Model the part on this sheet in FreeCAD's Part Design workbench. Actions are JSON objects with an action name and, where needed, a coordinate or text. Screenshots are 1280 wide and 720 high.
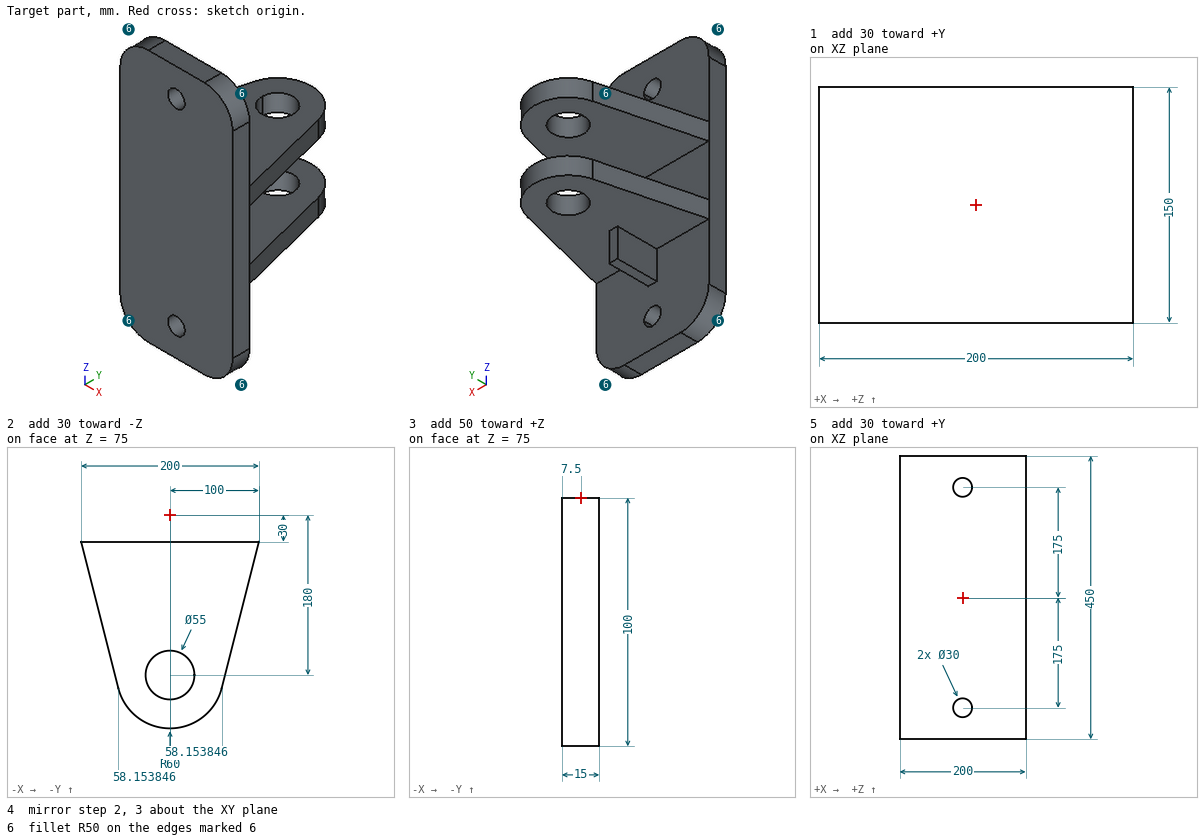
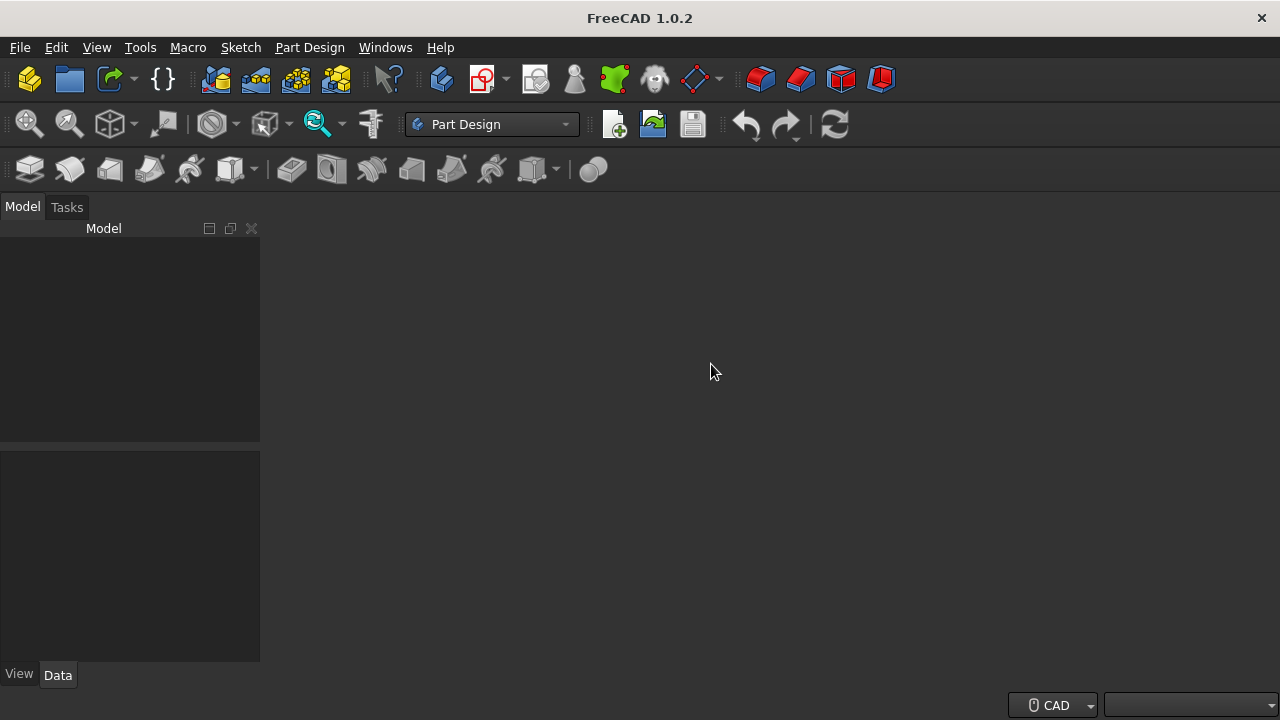
{"action": "left_click", "coordinate": [614, 124]}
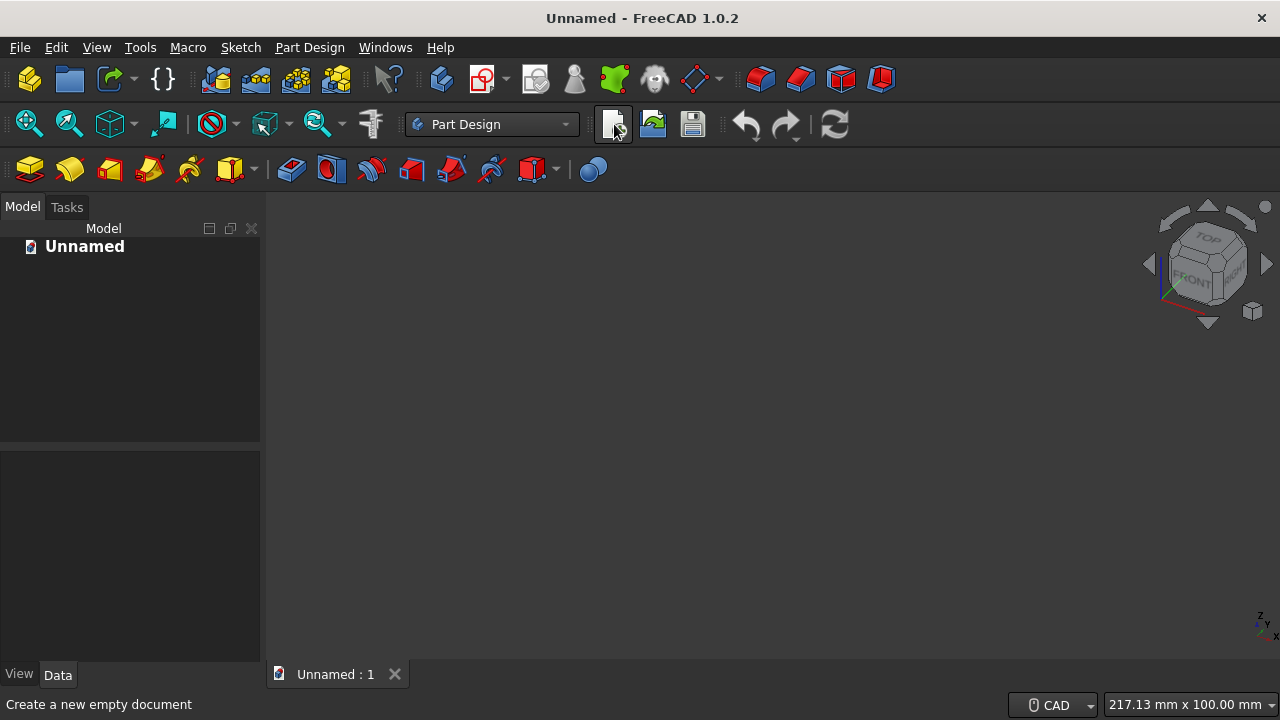
{"action": "left_click", "coordinate": [482, 80]}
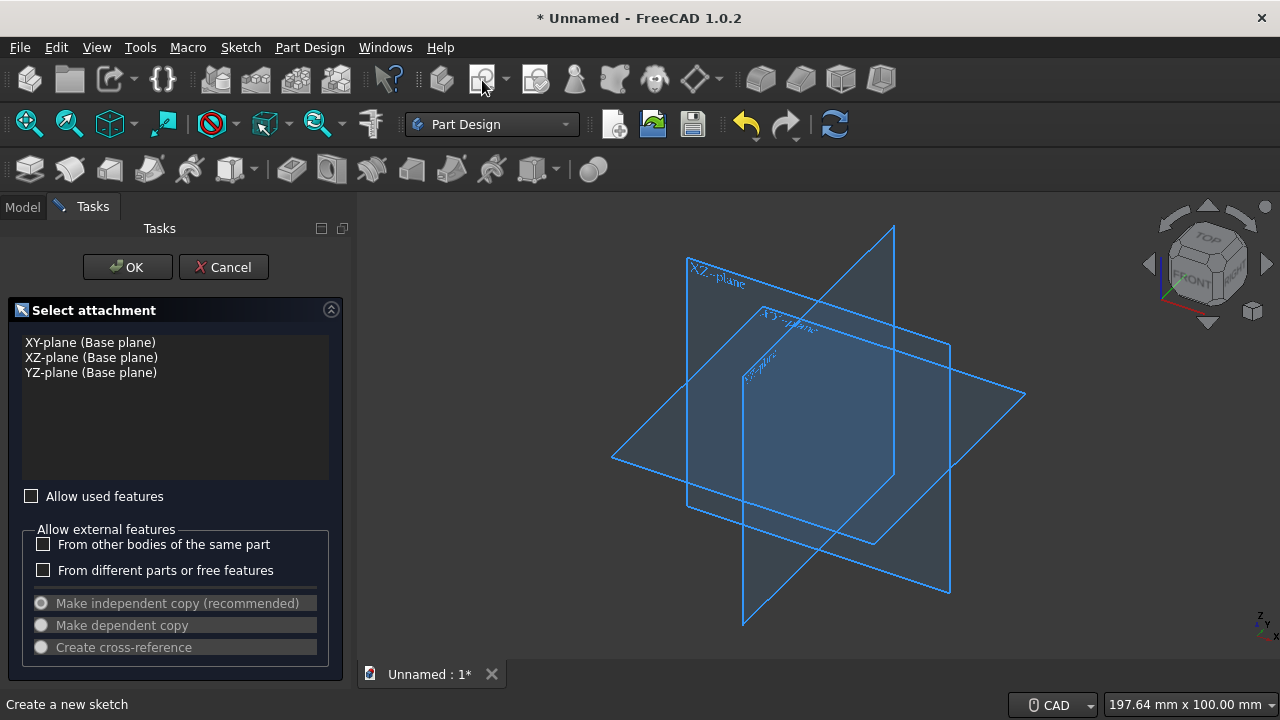
{"action": "left_click", "coordinate": [82, 358]}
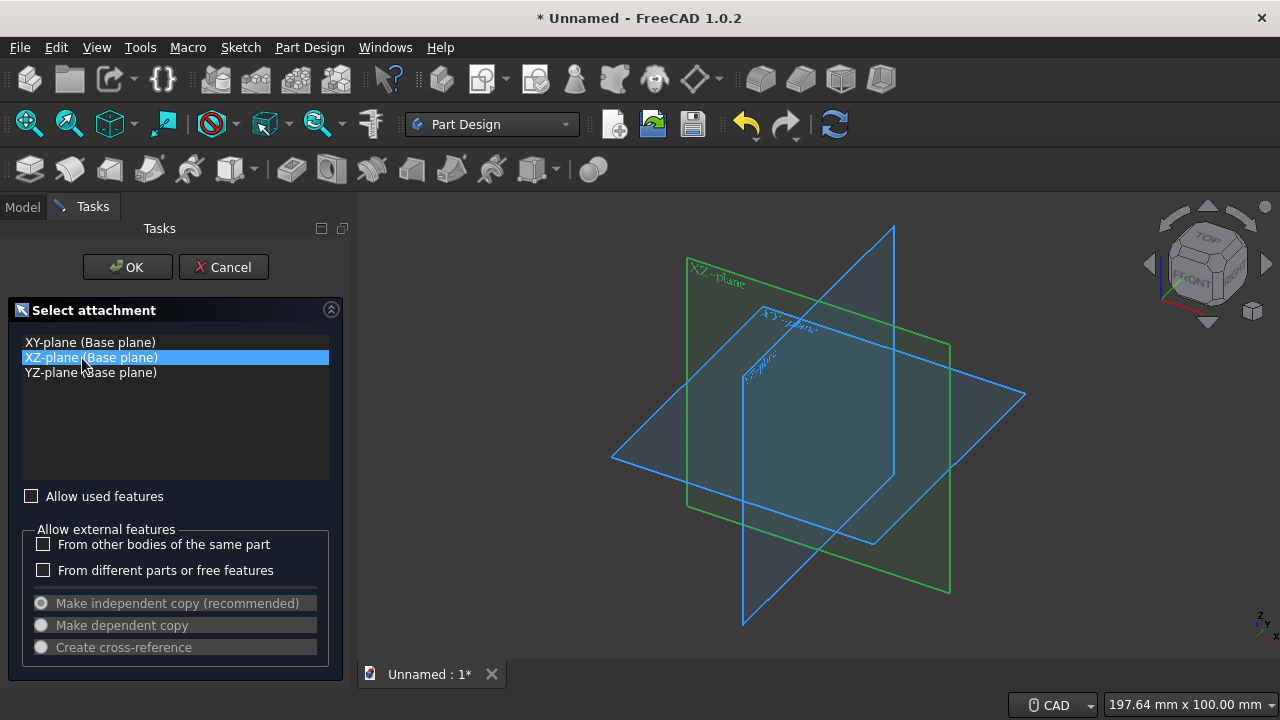
{"action": "left_click", "coordinate": [128, 267]}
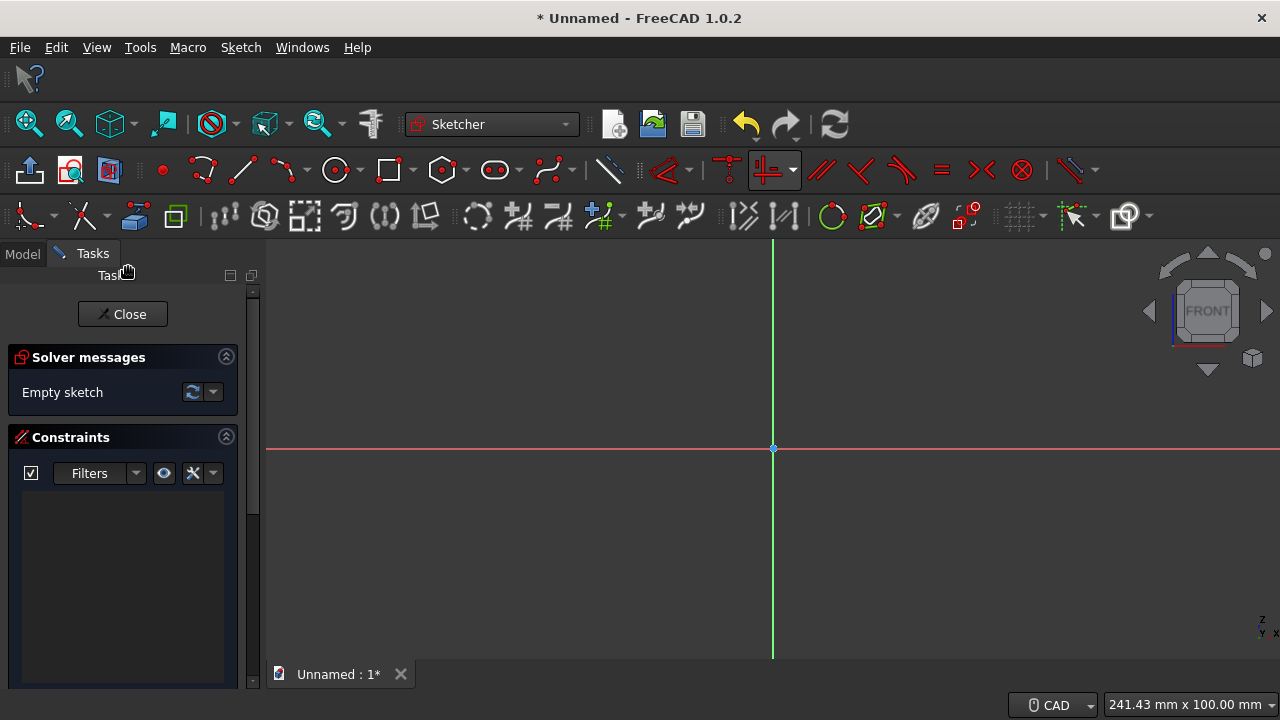
{"action": "scroll", "coordinate": [649, 449], "scroll_direction": "down", "scroll_amount": 4}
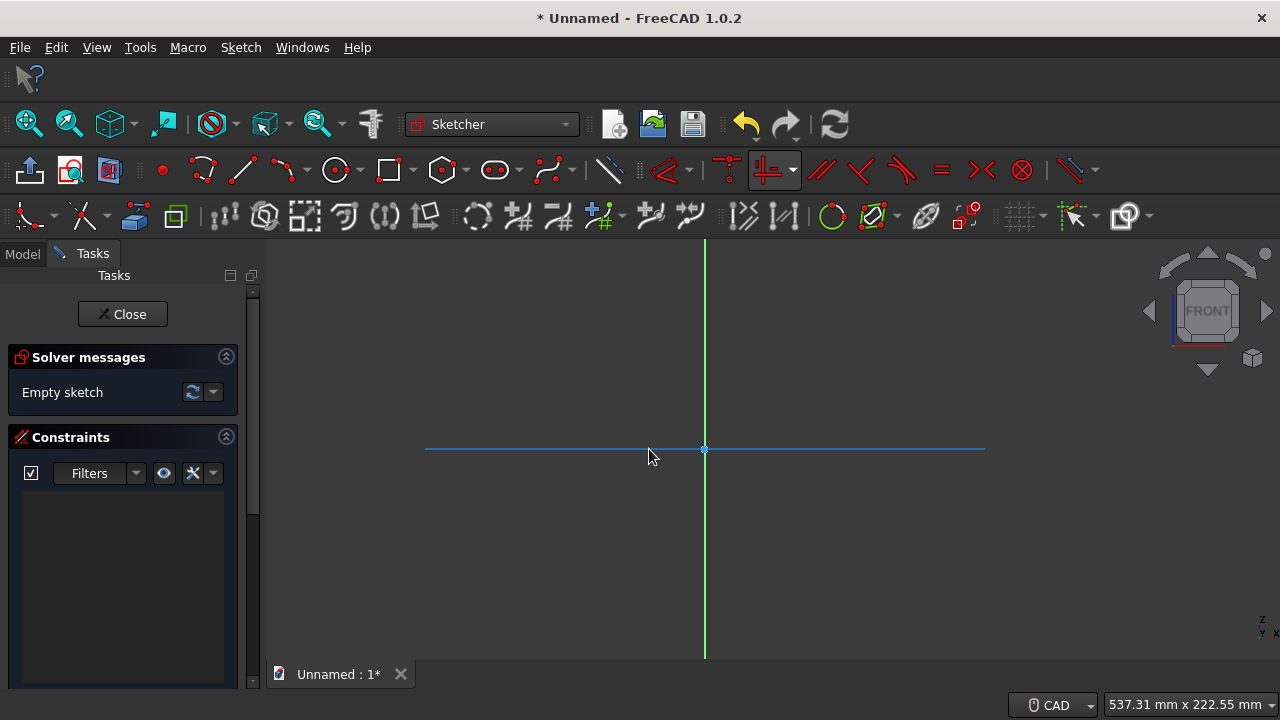
{"action": "left_click", "coordinate": [416, 170]}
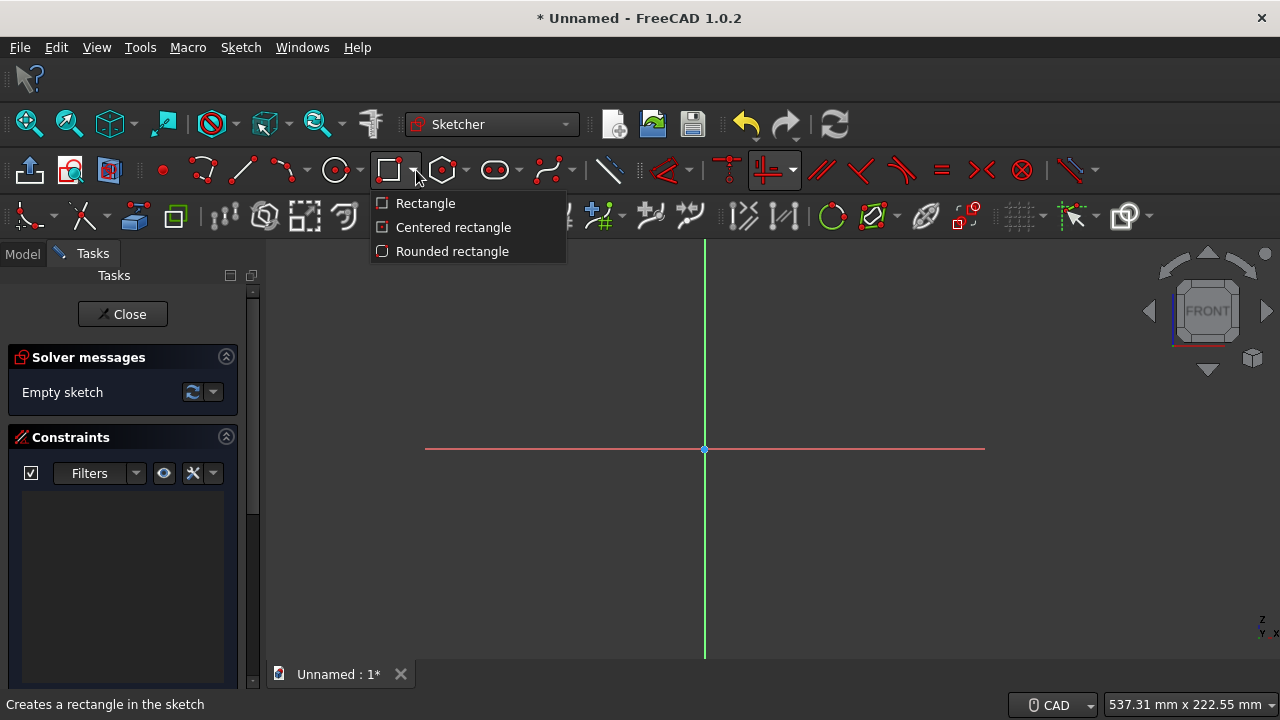
{"action": "left_click", "coordinate": [468, 227]}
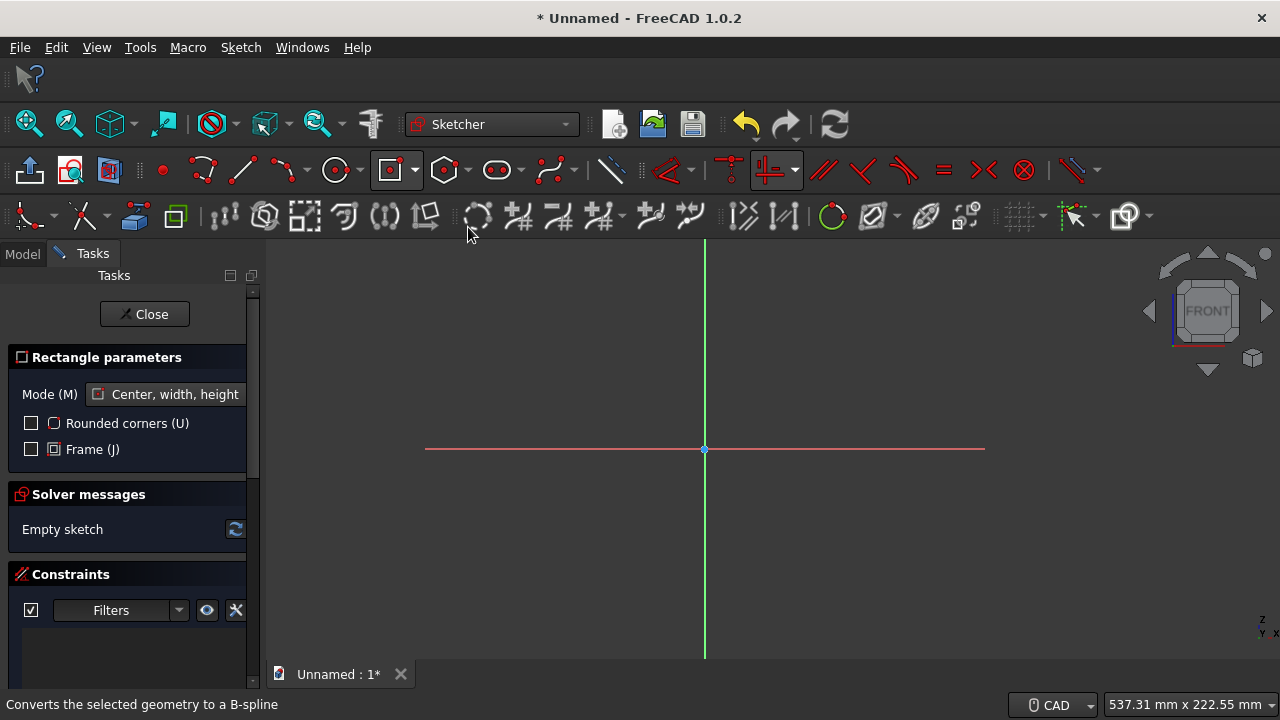
{"action": "left_click", "coordinate": [705, 449]}
{"action": "mouse_move", "coordinate": [894, 308]}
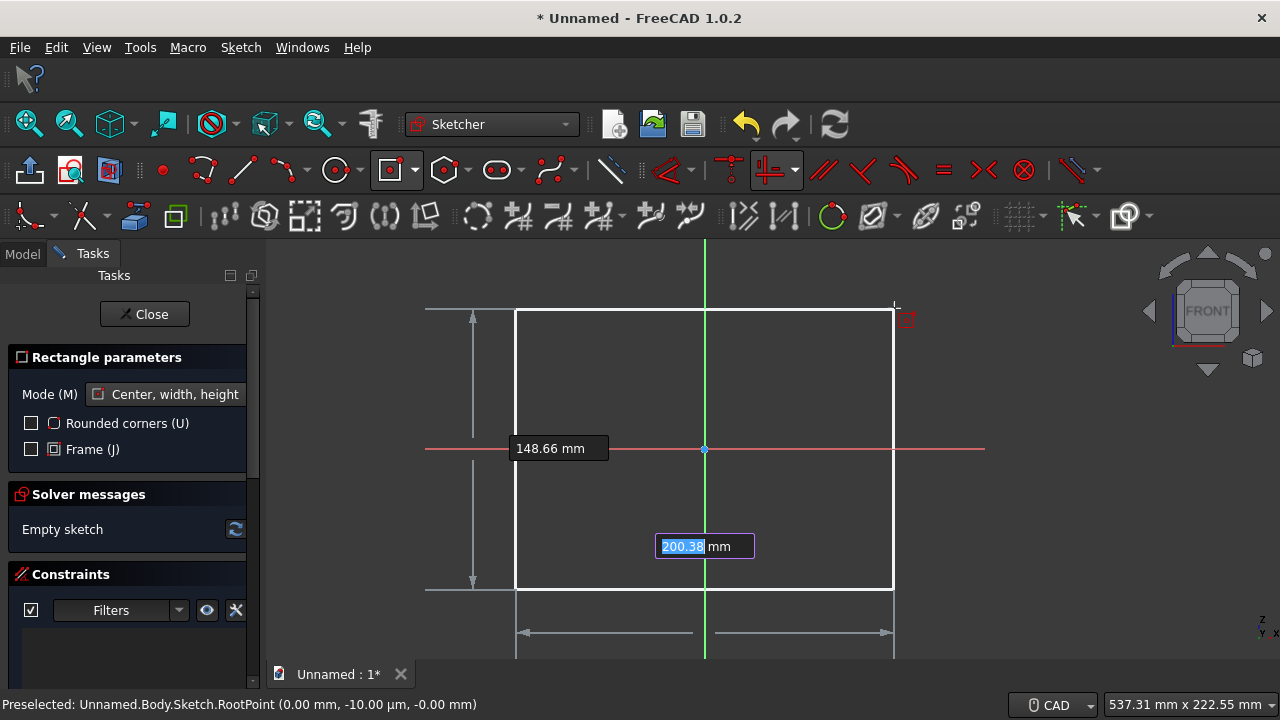
{"action": "type", "text": "200"}
{"action": "key", "text": "Tab"}
{"action": "type", "text": "150"}
{"action": "key", "text": "Return"}
{"action": "key", "text": "Escape"}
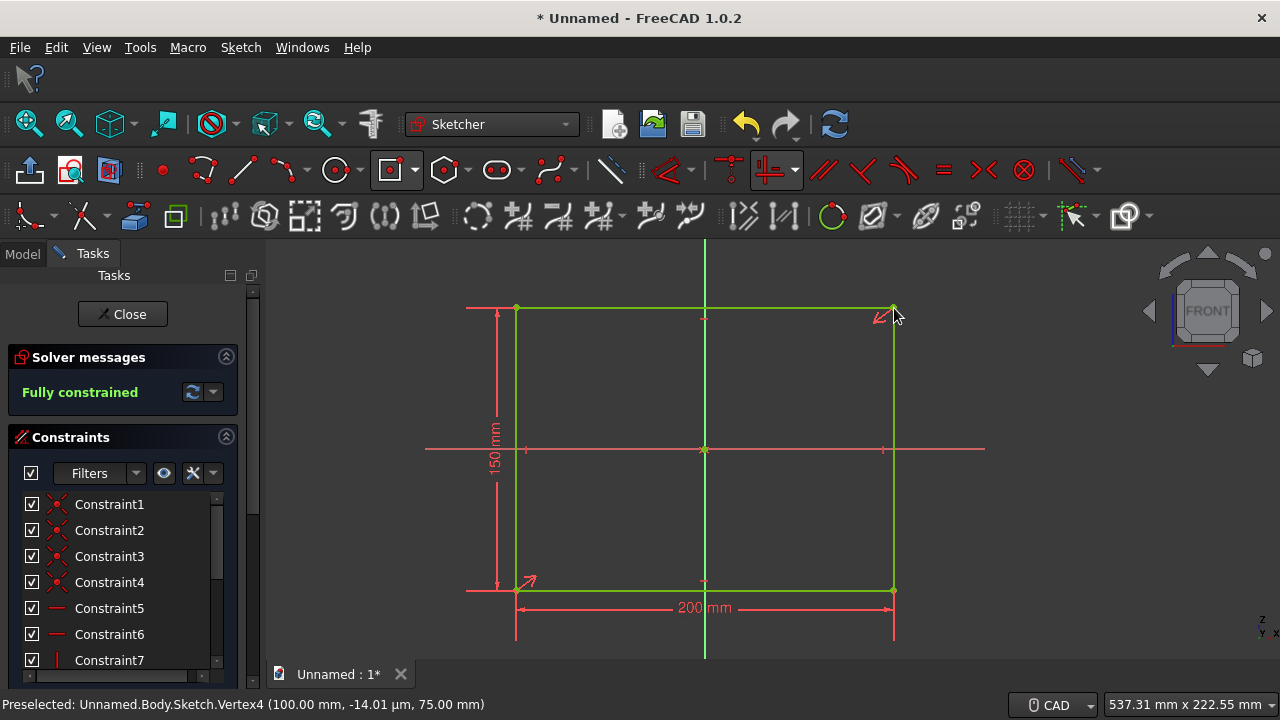
{"action": "left_click", "coordinate": [123, 314]}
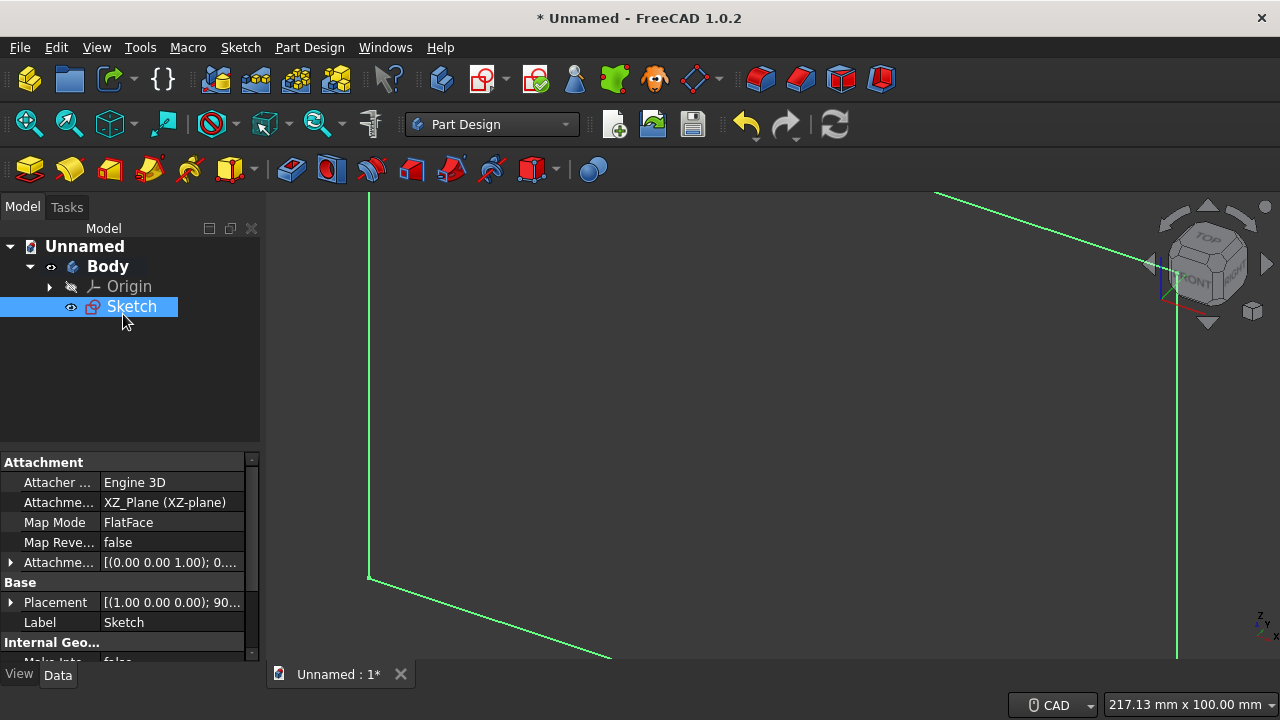
{"action": "left_click", "coordinate": [30, 170]}